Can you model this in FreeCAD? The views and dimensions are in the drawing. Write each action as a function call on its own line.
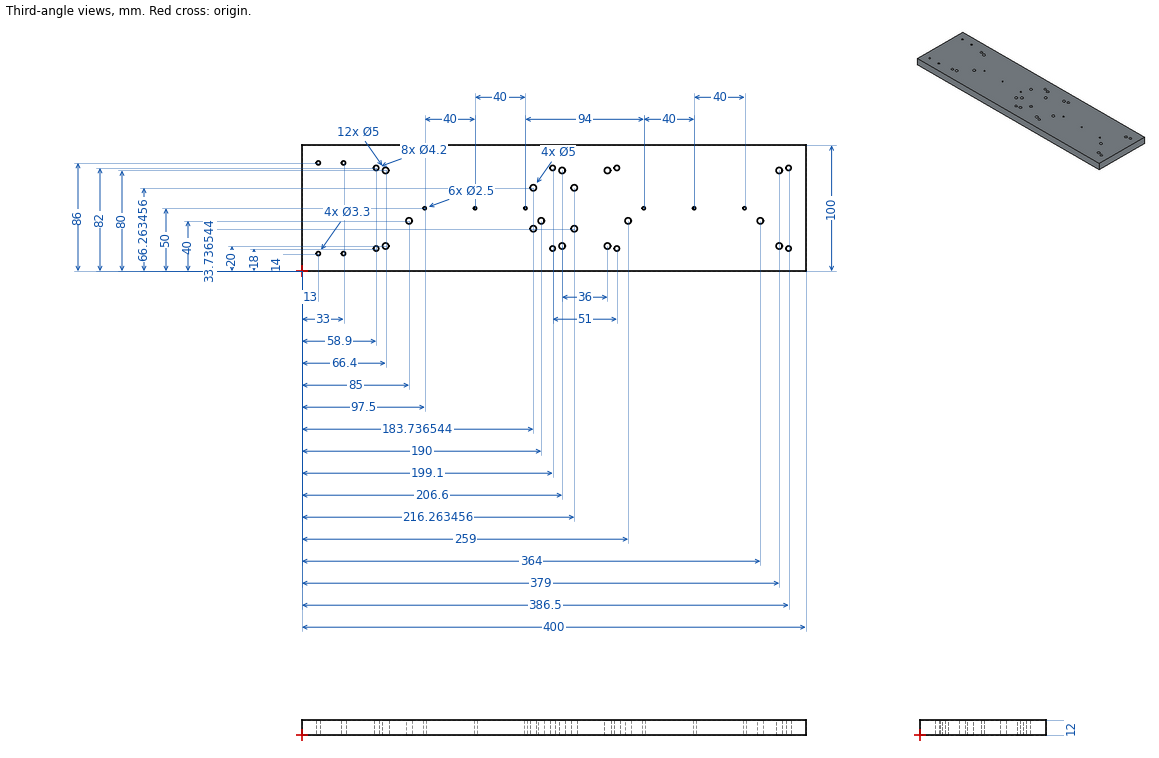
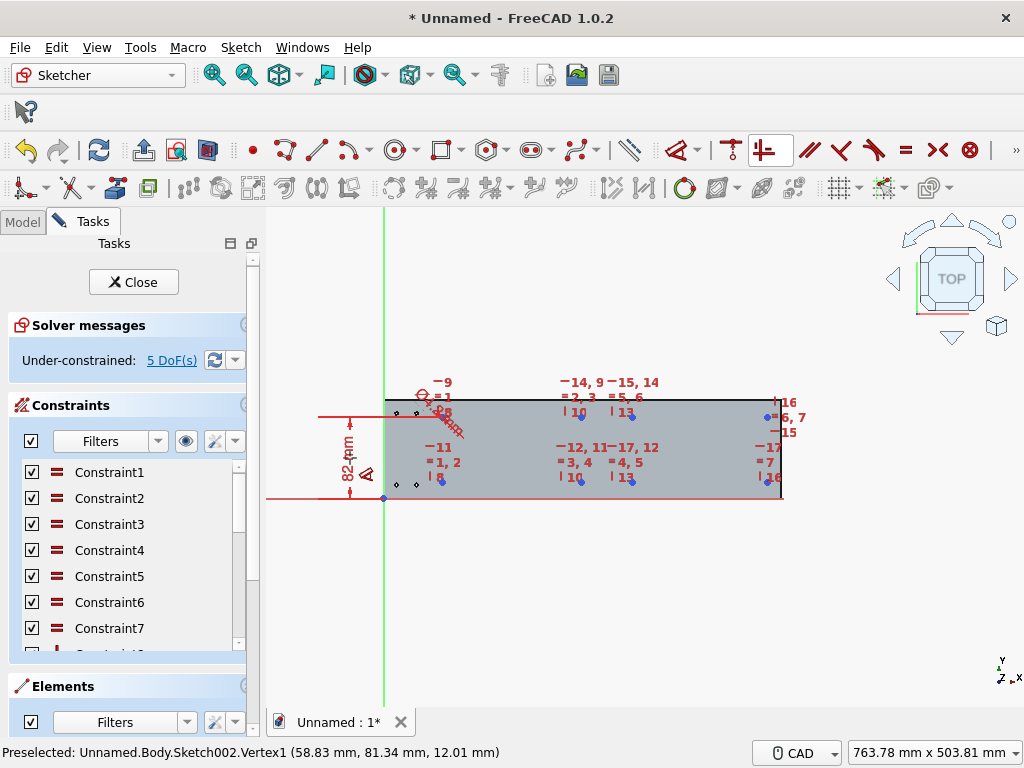
scroll(442, 482, up, 4)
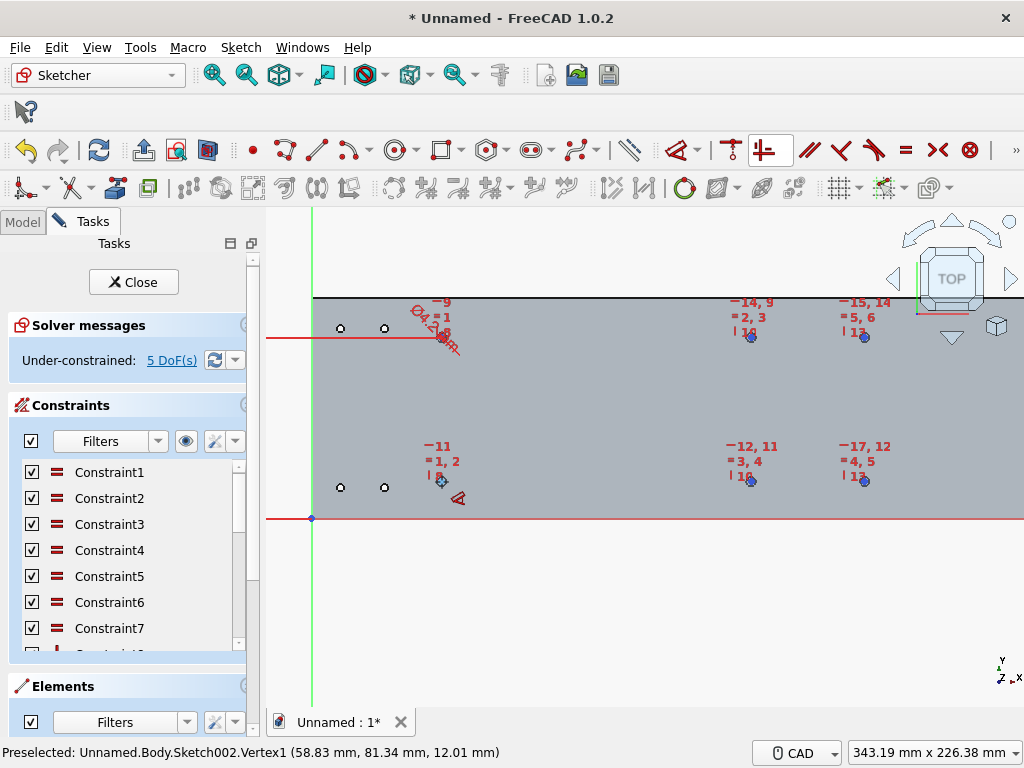
click(442, 482)
click(476, 500)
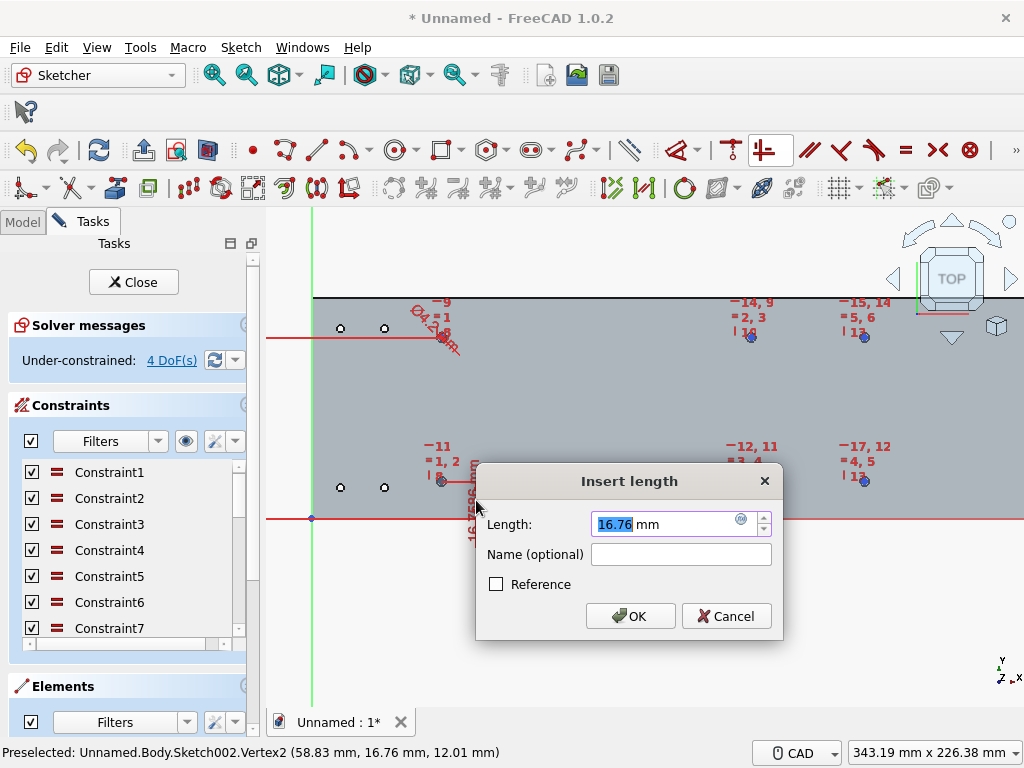
text(18)
key(Return)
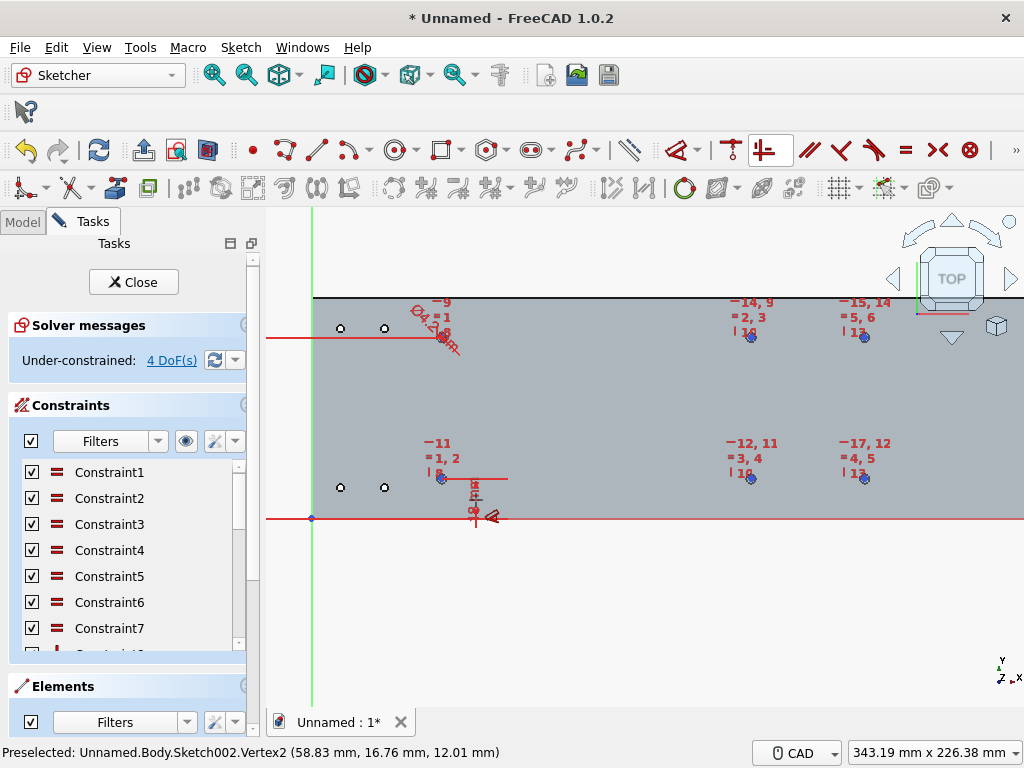
click(751, 479)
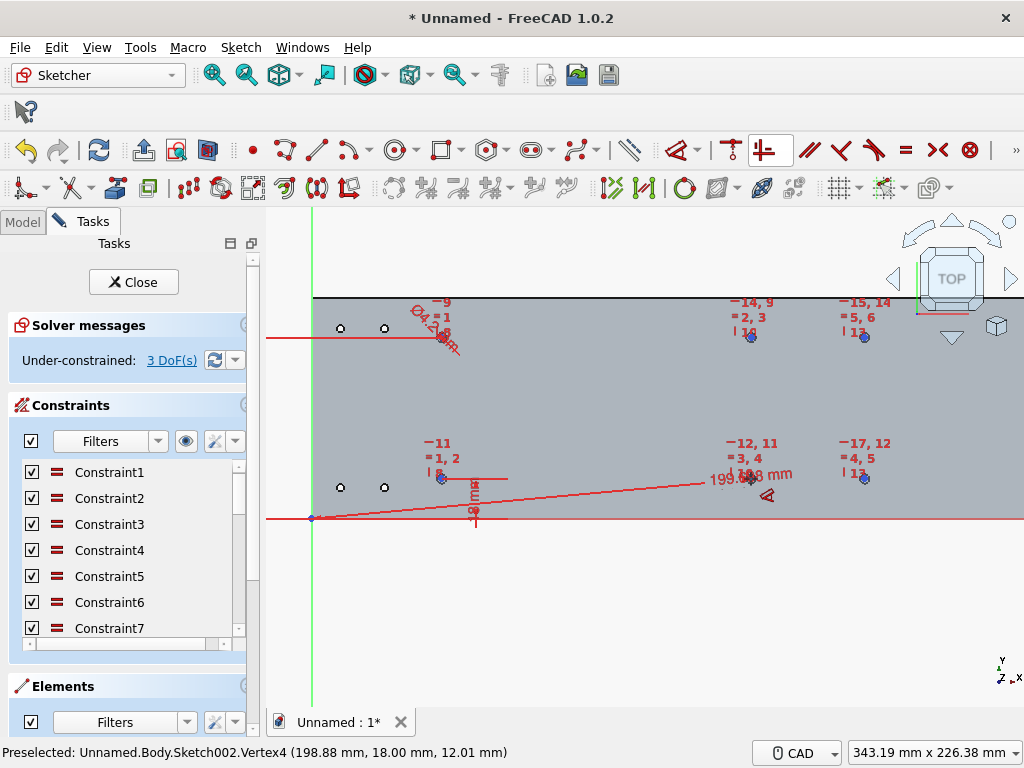
scroll(442, 482, down, 4)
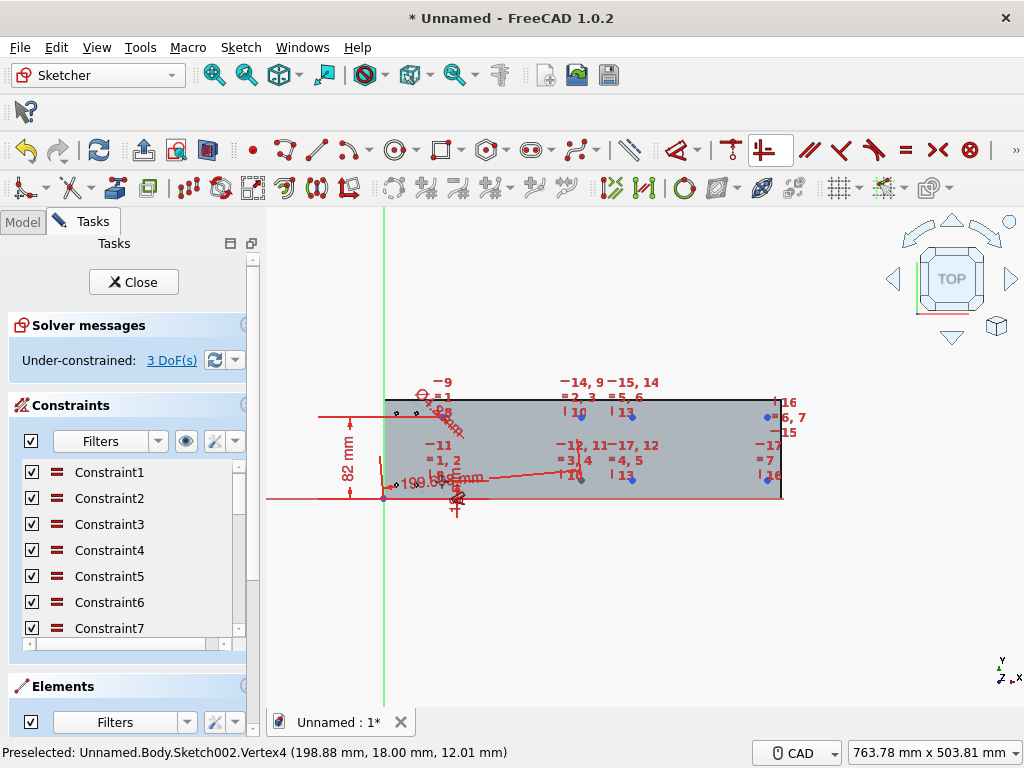
click(632, 481)
click(607, 515)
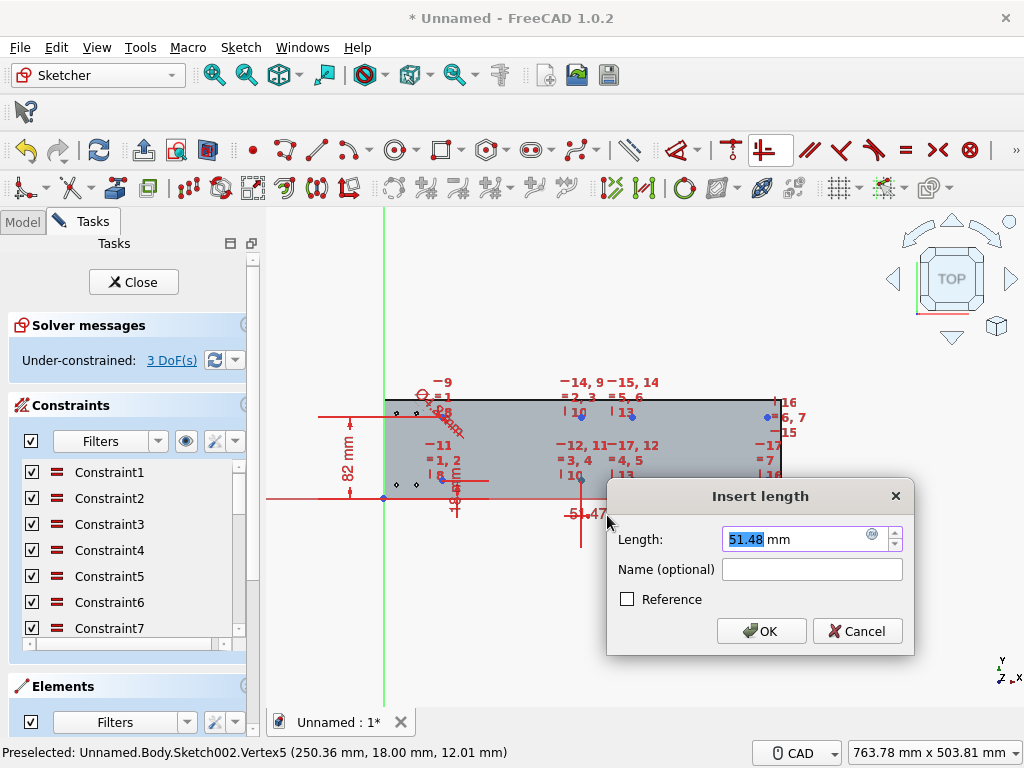
text(51)
key(Return)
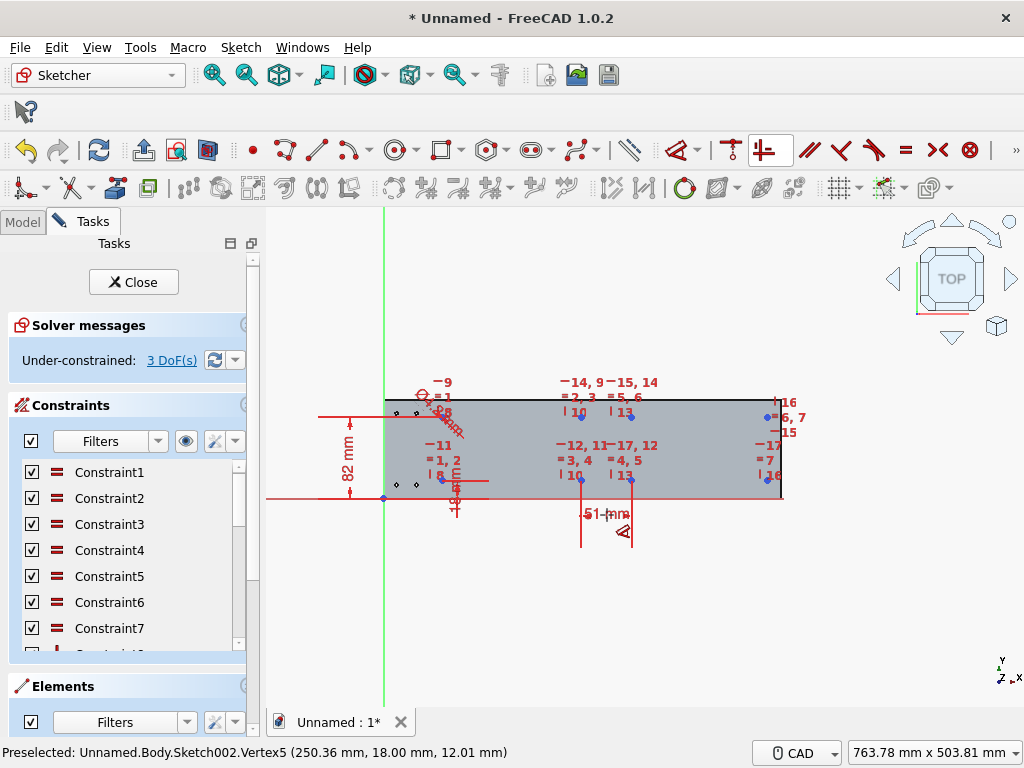
click(442, 417)
click(413, 533)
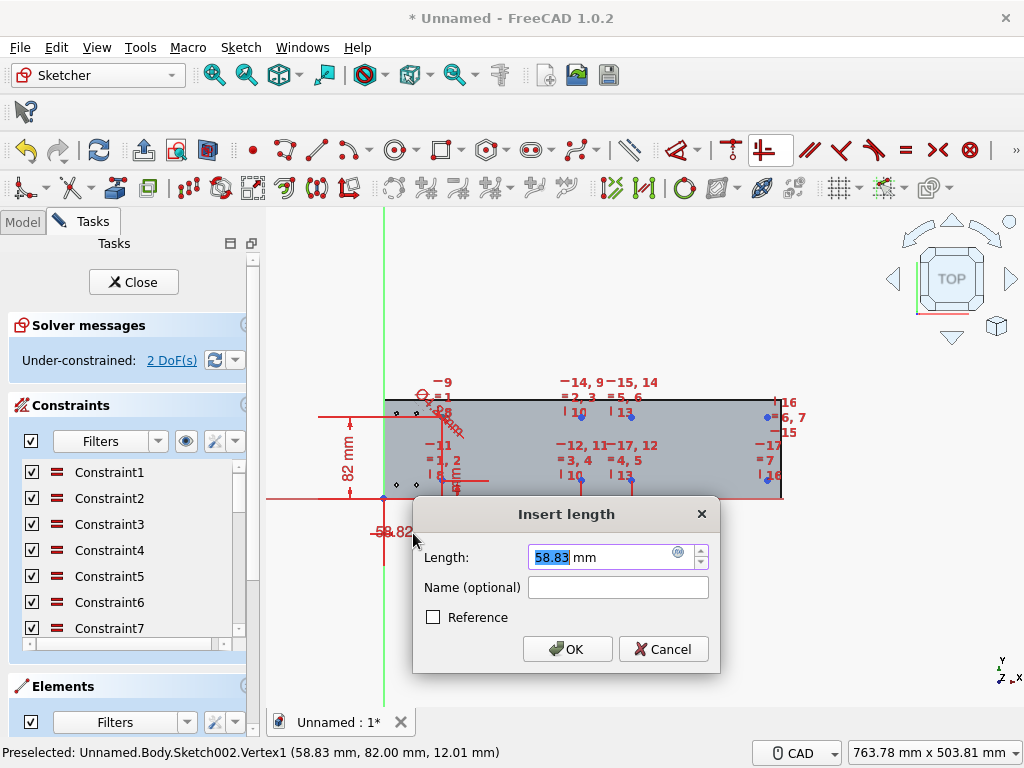
text(58.9)
key(Return)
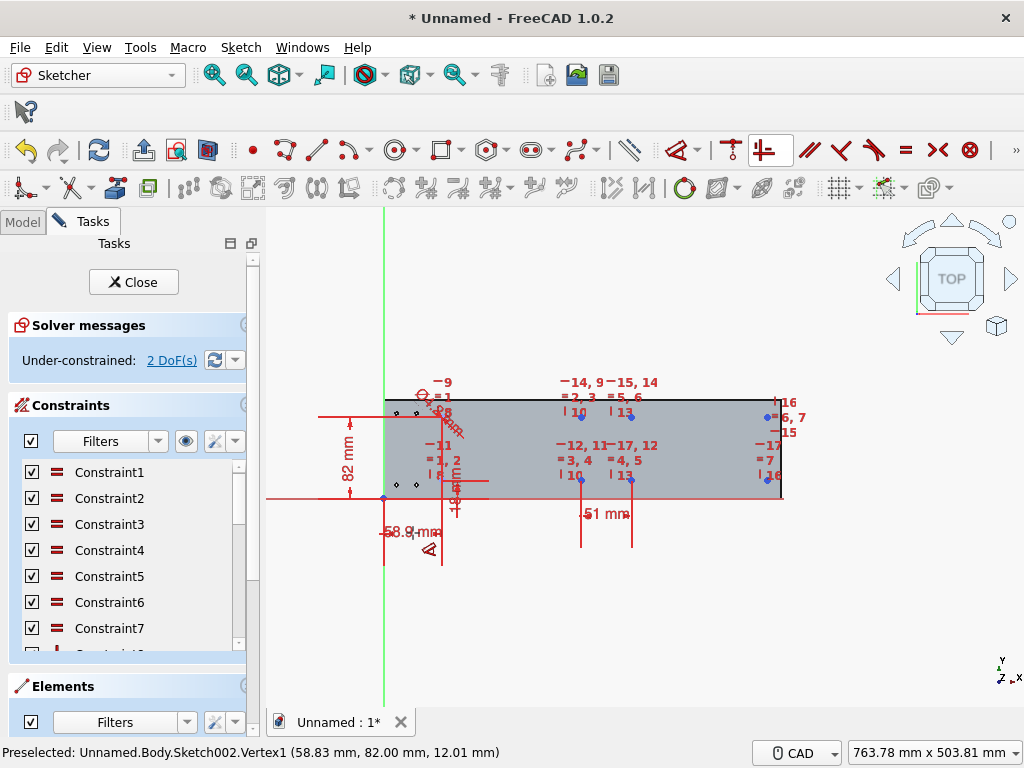
click(581, 417)
click(528, 533)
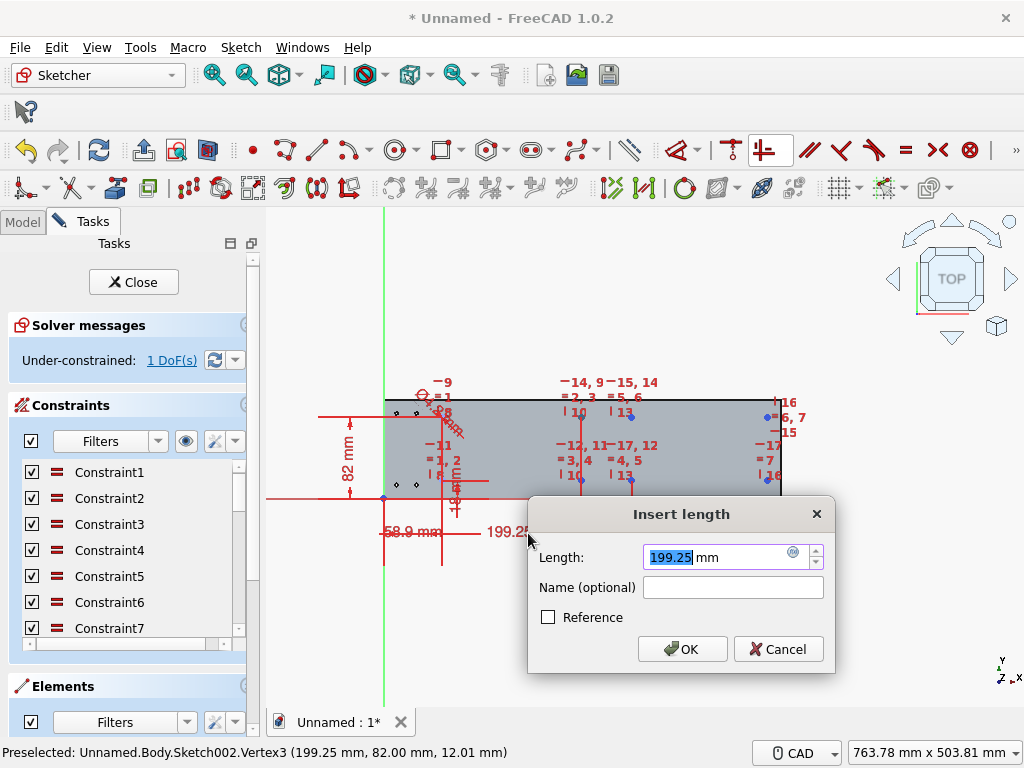
text(199.1)
key(Return)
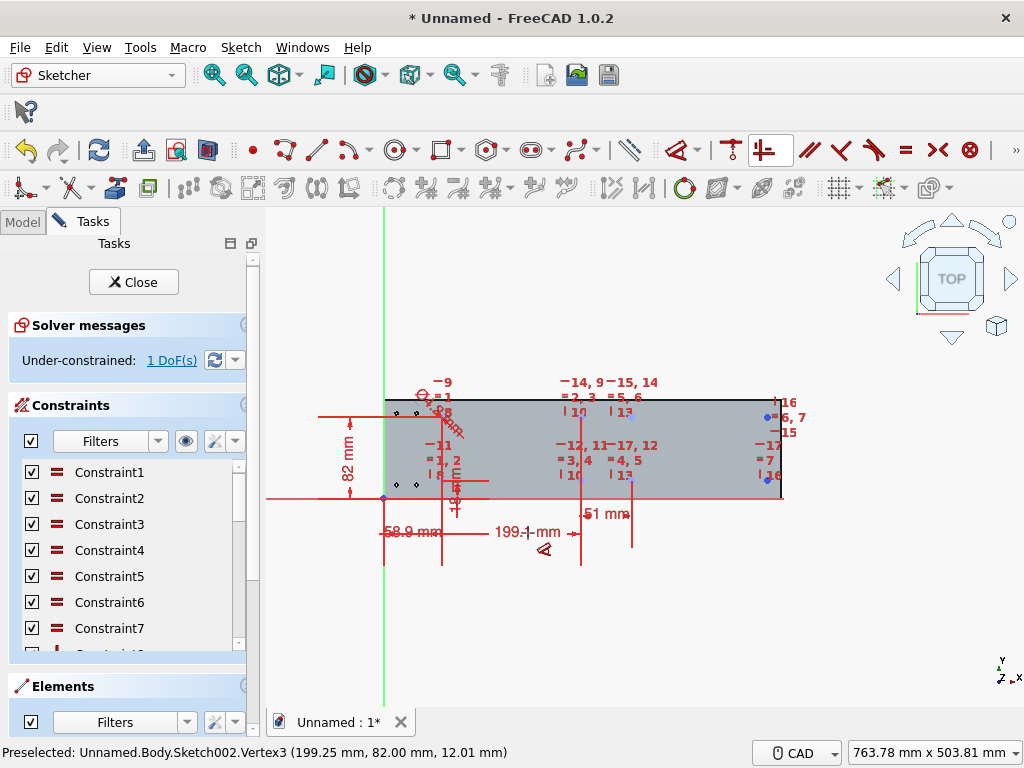
click(767, 417)
click(710, 533)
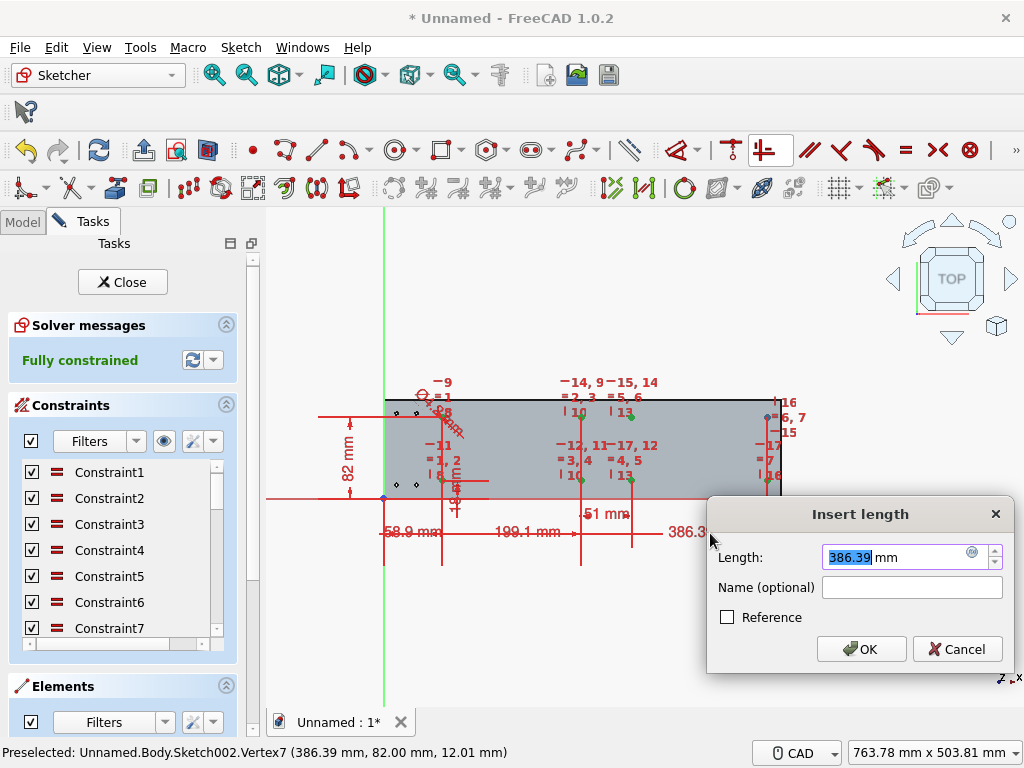
text(386.5)
key(Return)
key(Escape)